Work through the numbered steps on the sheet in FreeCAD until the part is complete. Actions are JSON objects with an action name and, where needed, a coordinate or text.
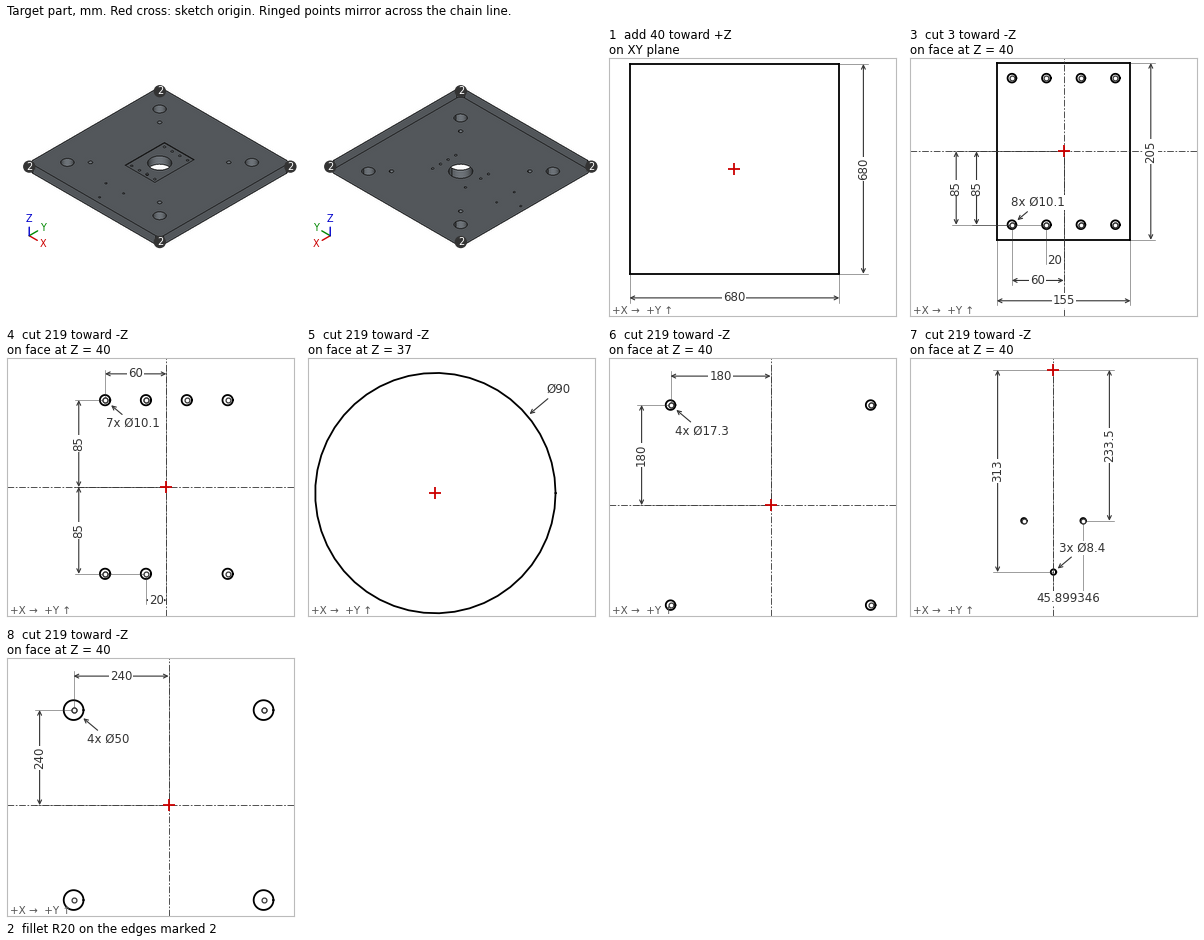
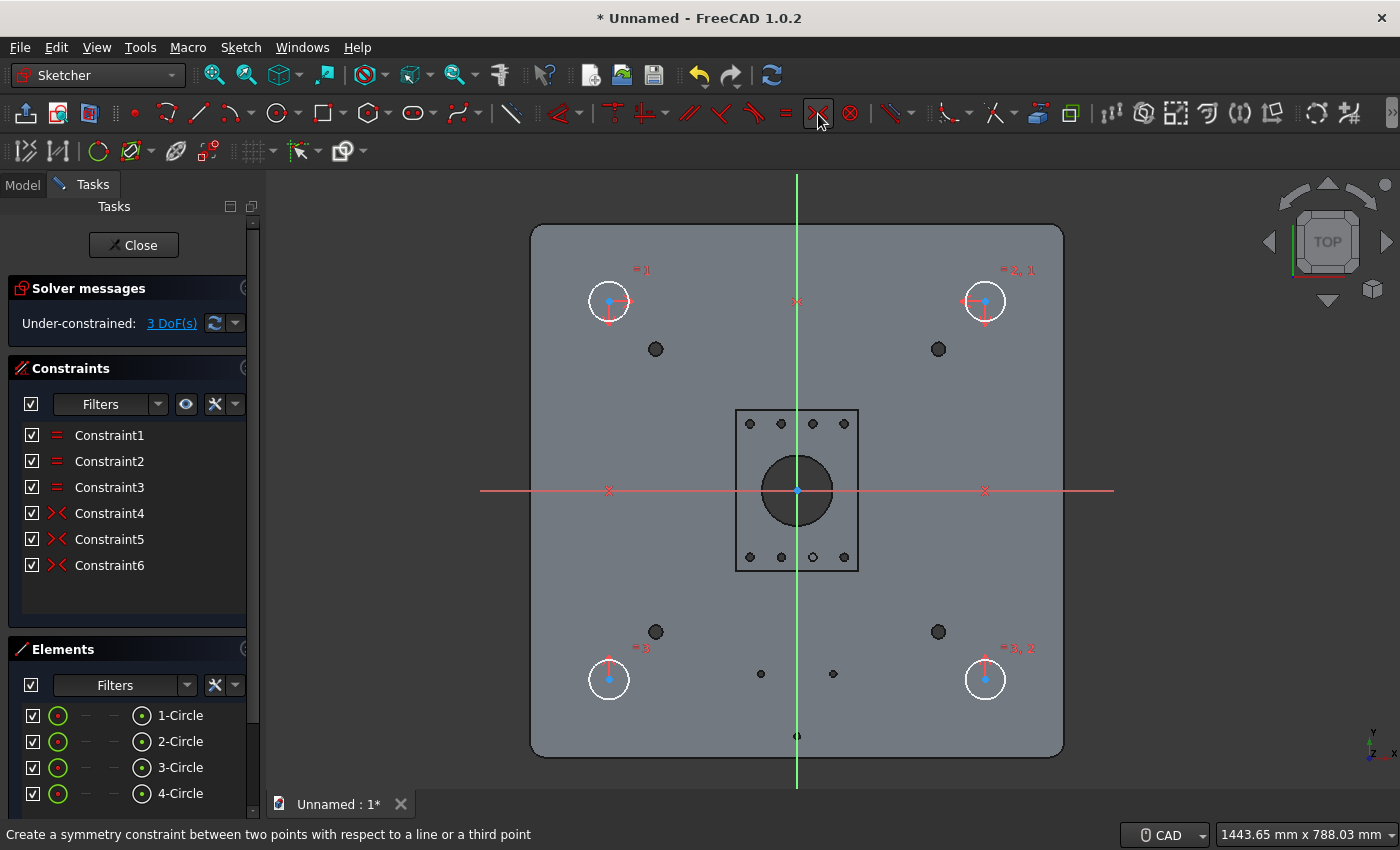
{"action": "left_click", "coordinate": [558, 114]}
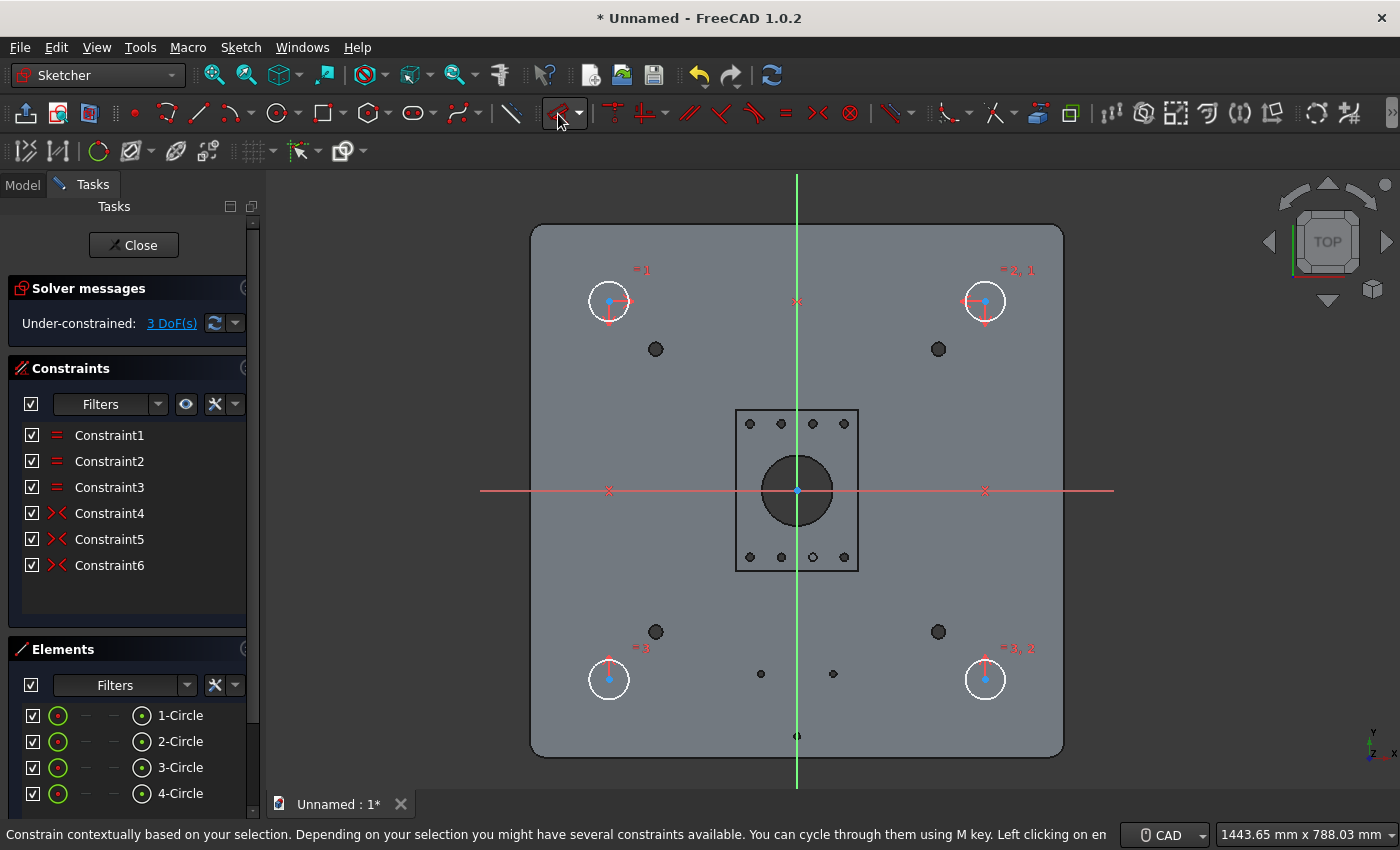
{"action": "left_click", "coordinate": [623, 288]}
{"action": "left_click", "coordinate": [646, 266]}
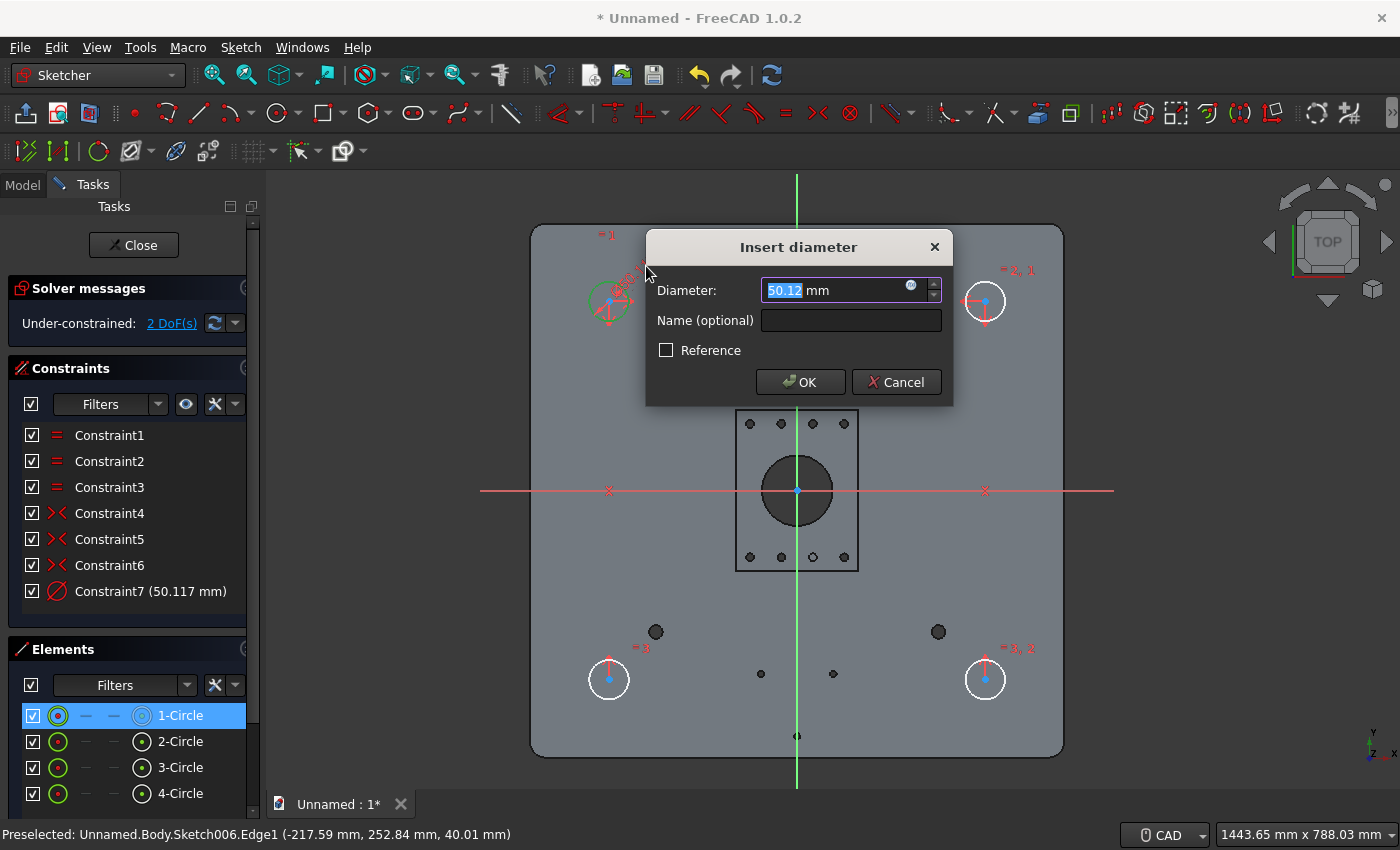
{"action": "type", "text": "50"}
{"action": "key", "text": "Return"}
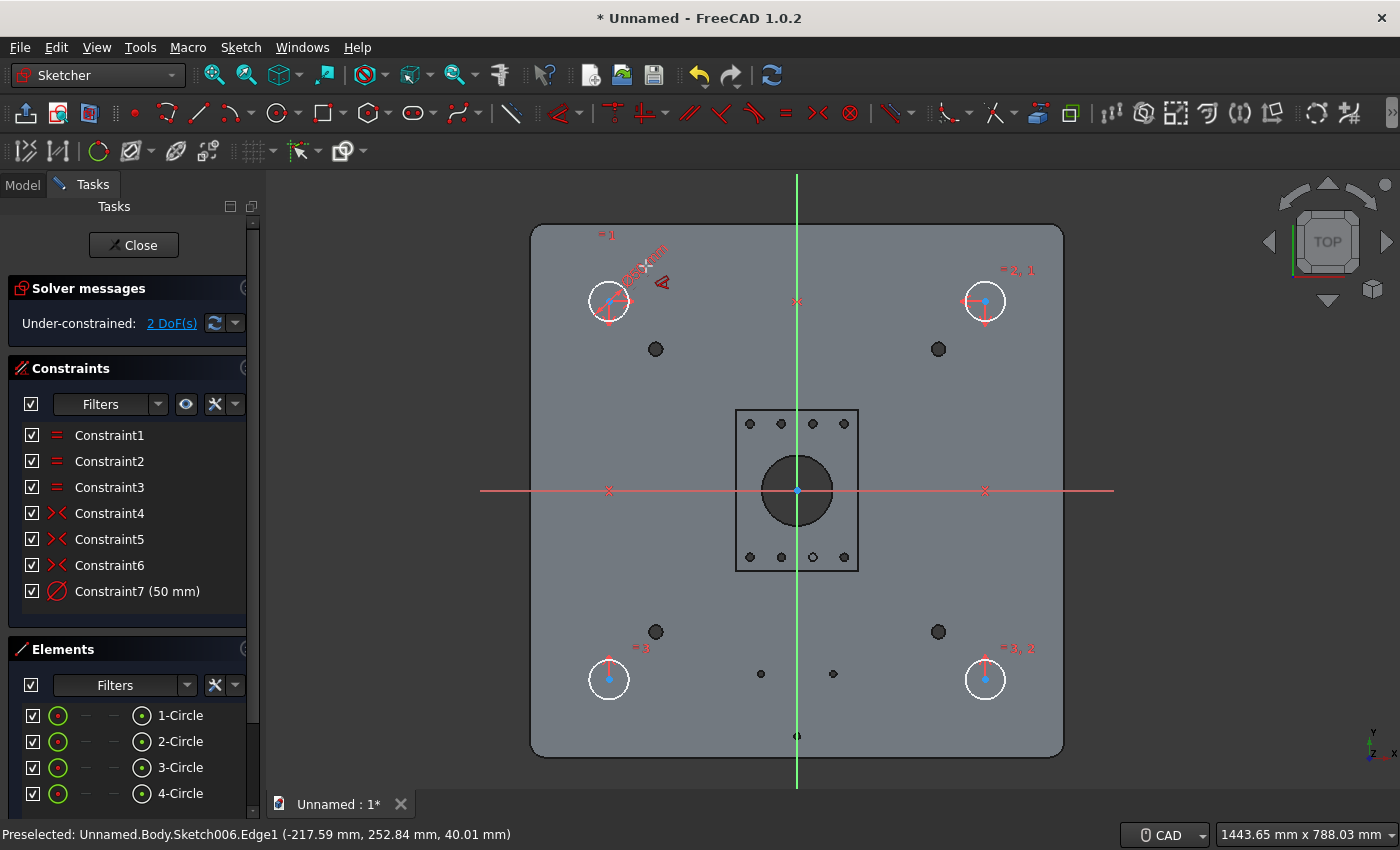
{"action": "left_click", "coordinate": [609, 301]}
{"action": "left_click", "coordinate": [746, 267]}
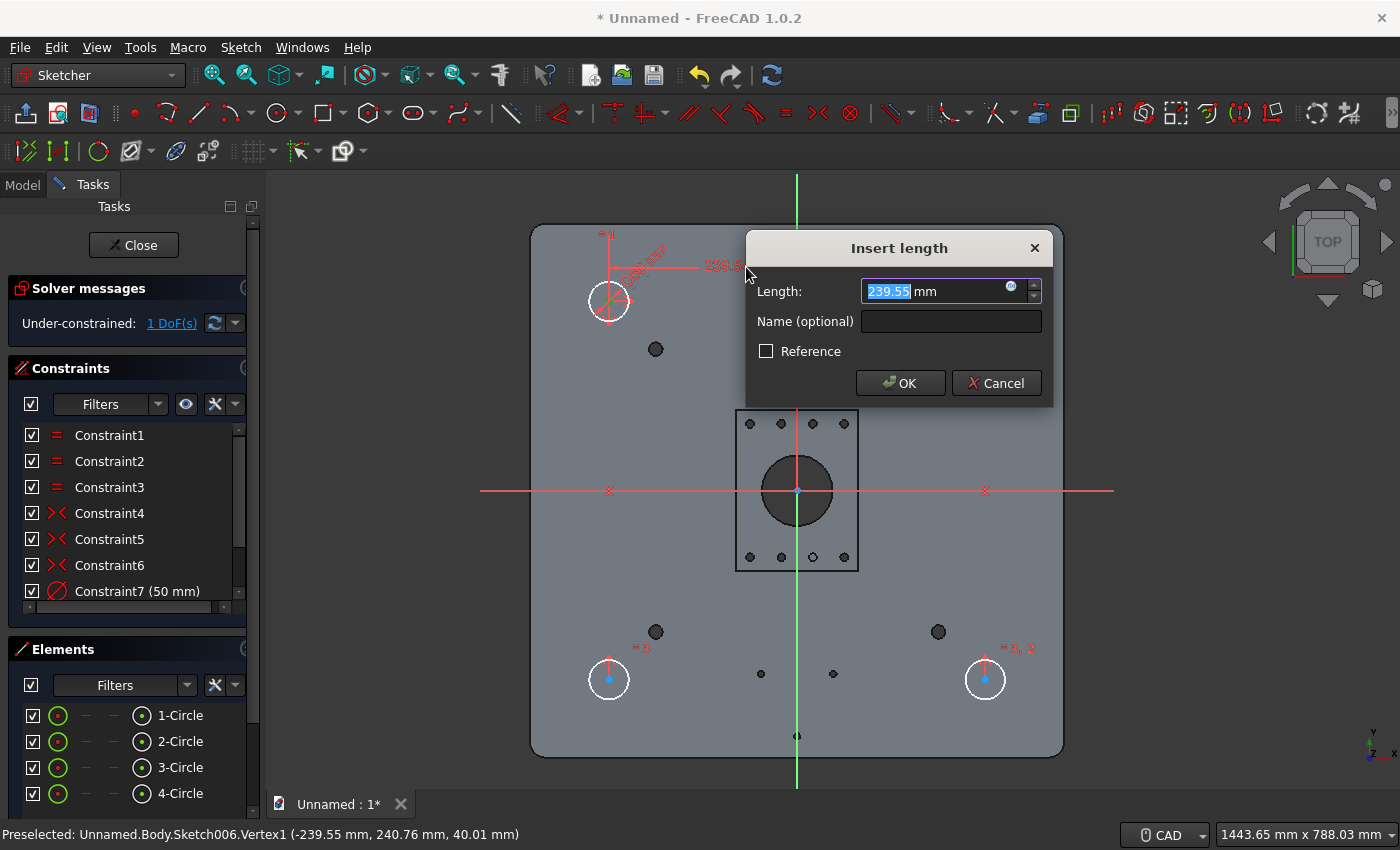
{"action": "type", "text": "240"}
{"action": "key", "text": "Return"}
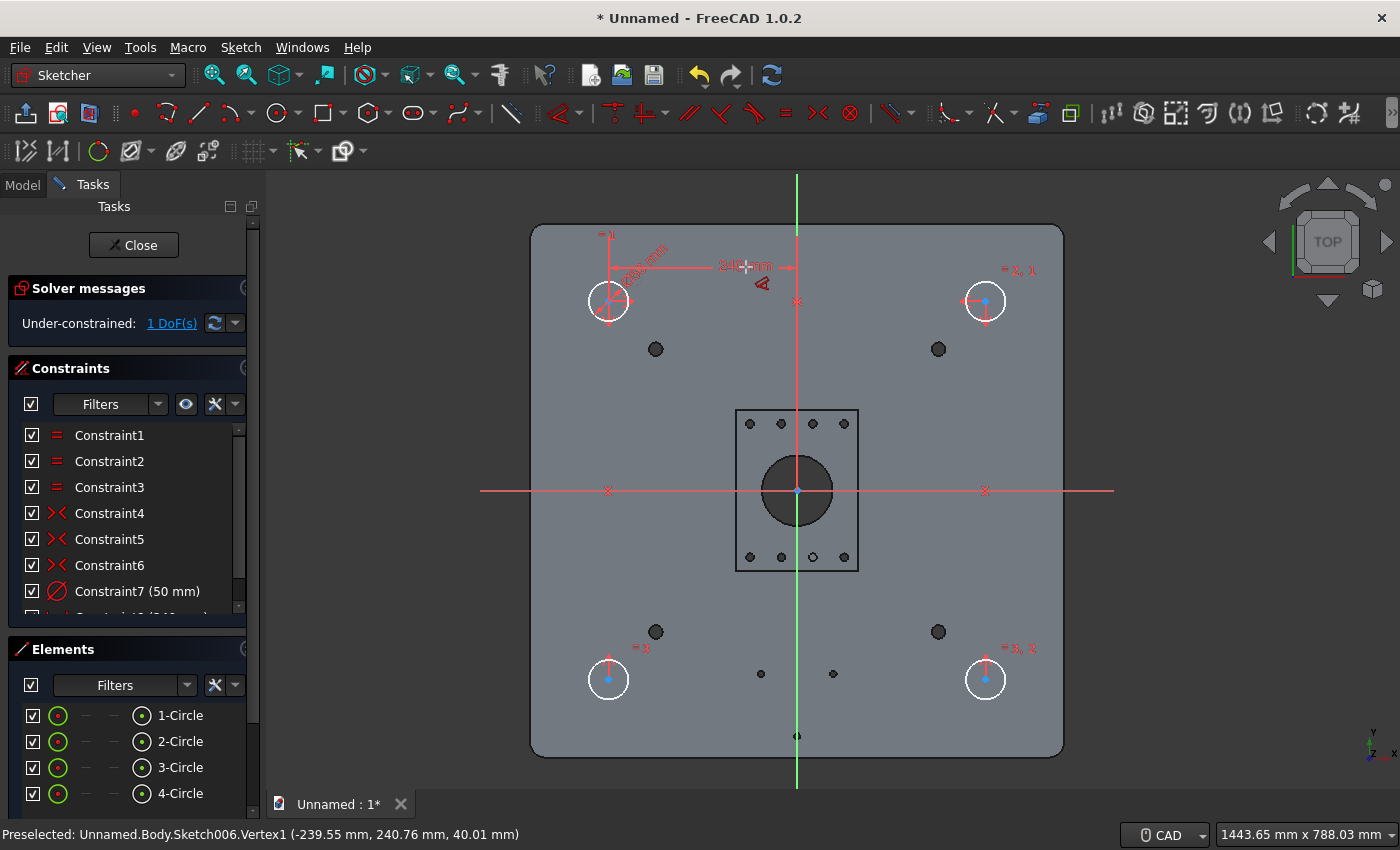
{"action": "left_click", "coordinate": [609, 301]}
{"action": "left_click", "coordinate": [575, 396]}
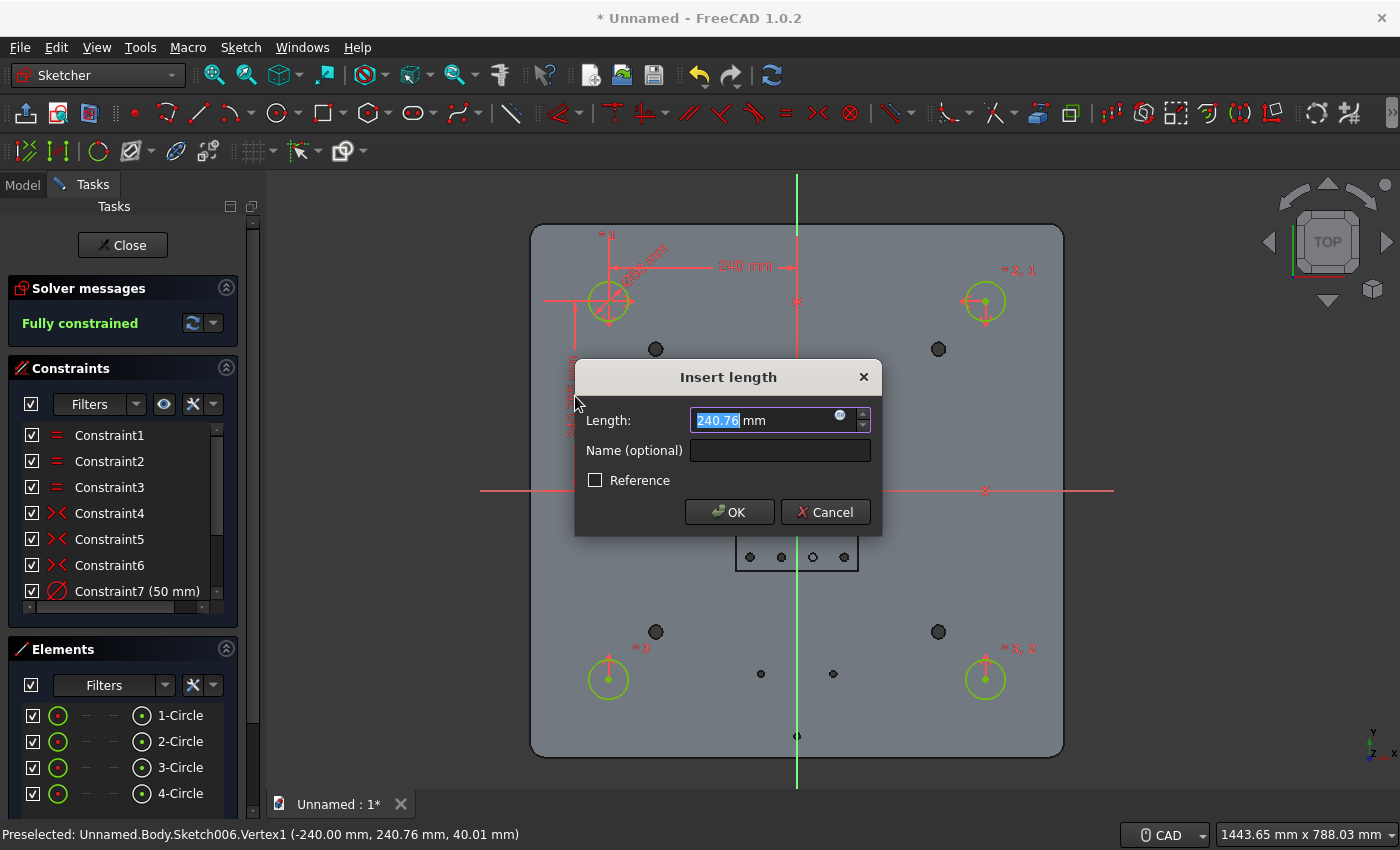
{"action": "type", "text": "240"}
{"action": "key", "text": "Return"}
{"action": "key", "text": "Escape"}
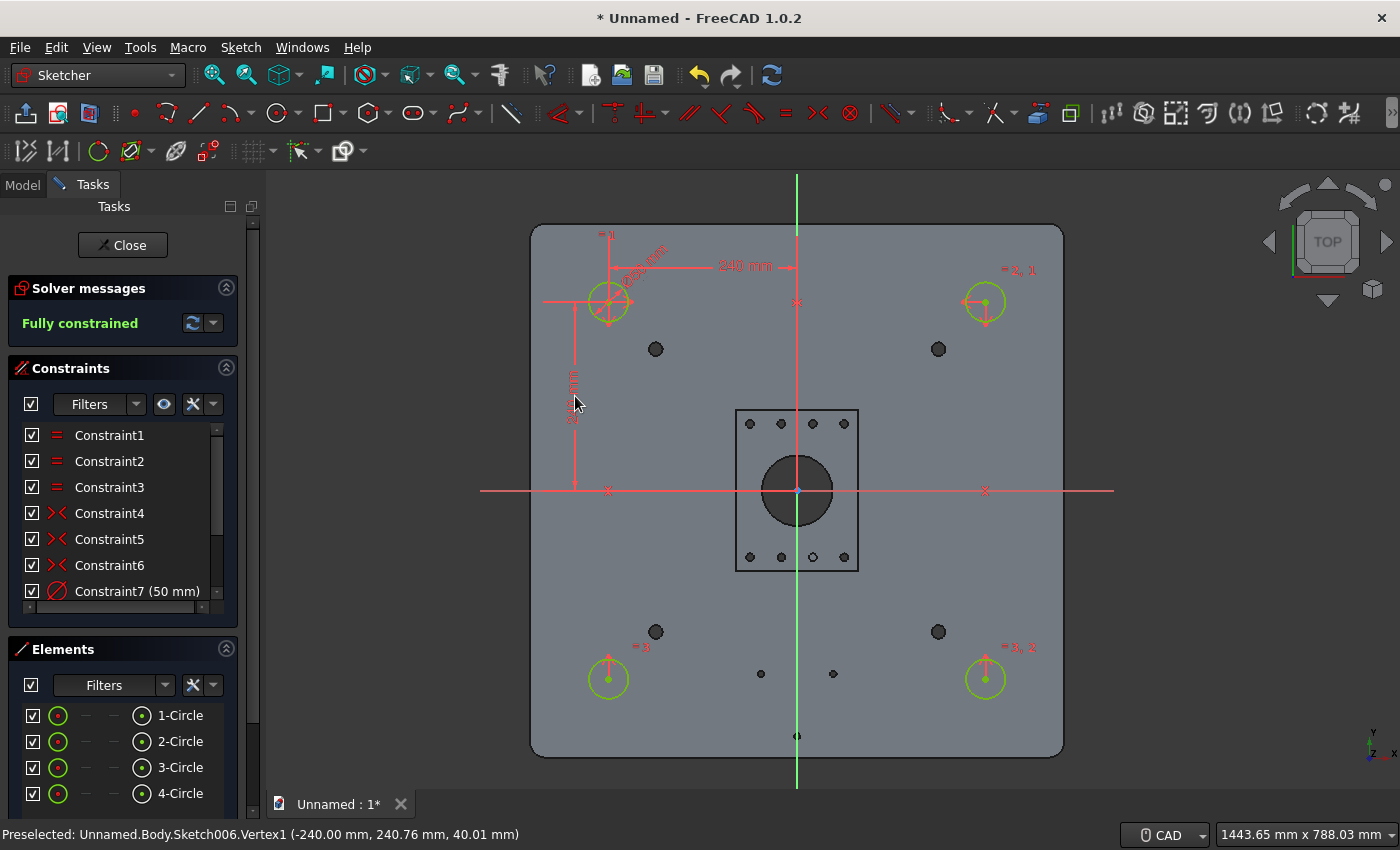
{"action": "left_click", "coordinate": [123, 245]}